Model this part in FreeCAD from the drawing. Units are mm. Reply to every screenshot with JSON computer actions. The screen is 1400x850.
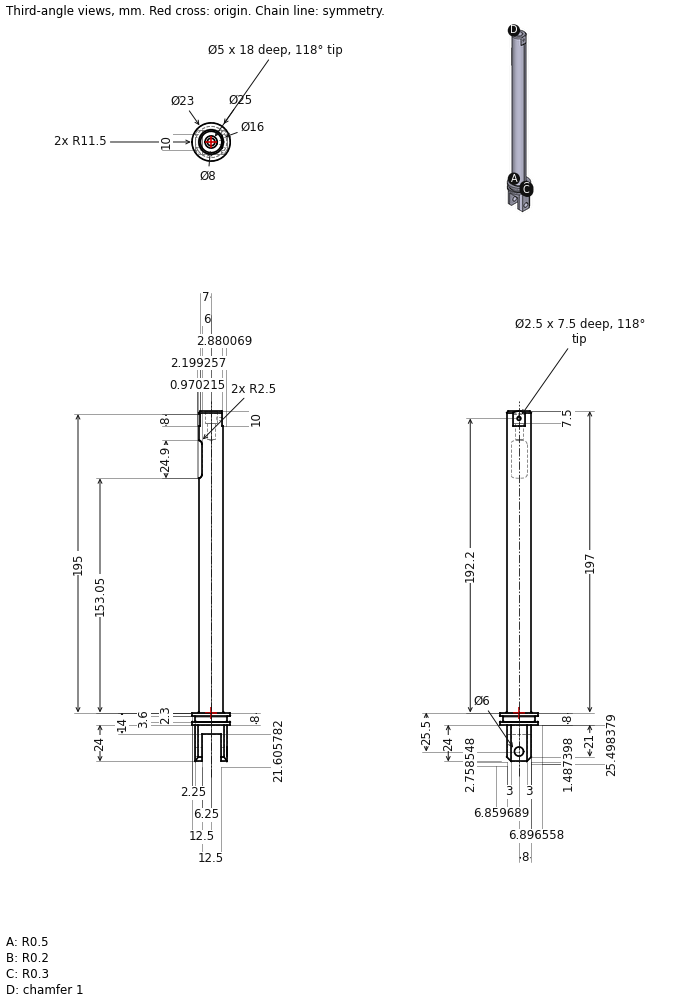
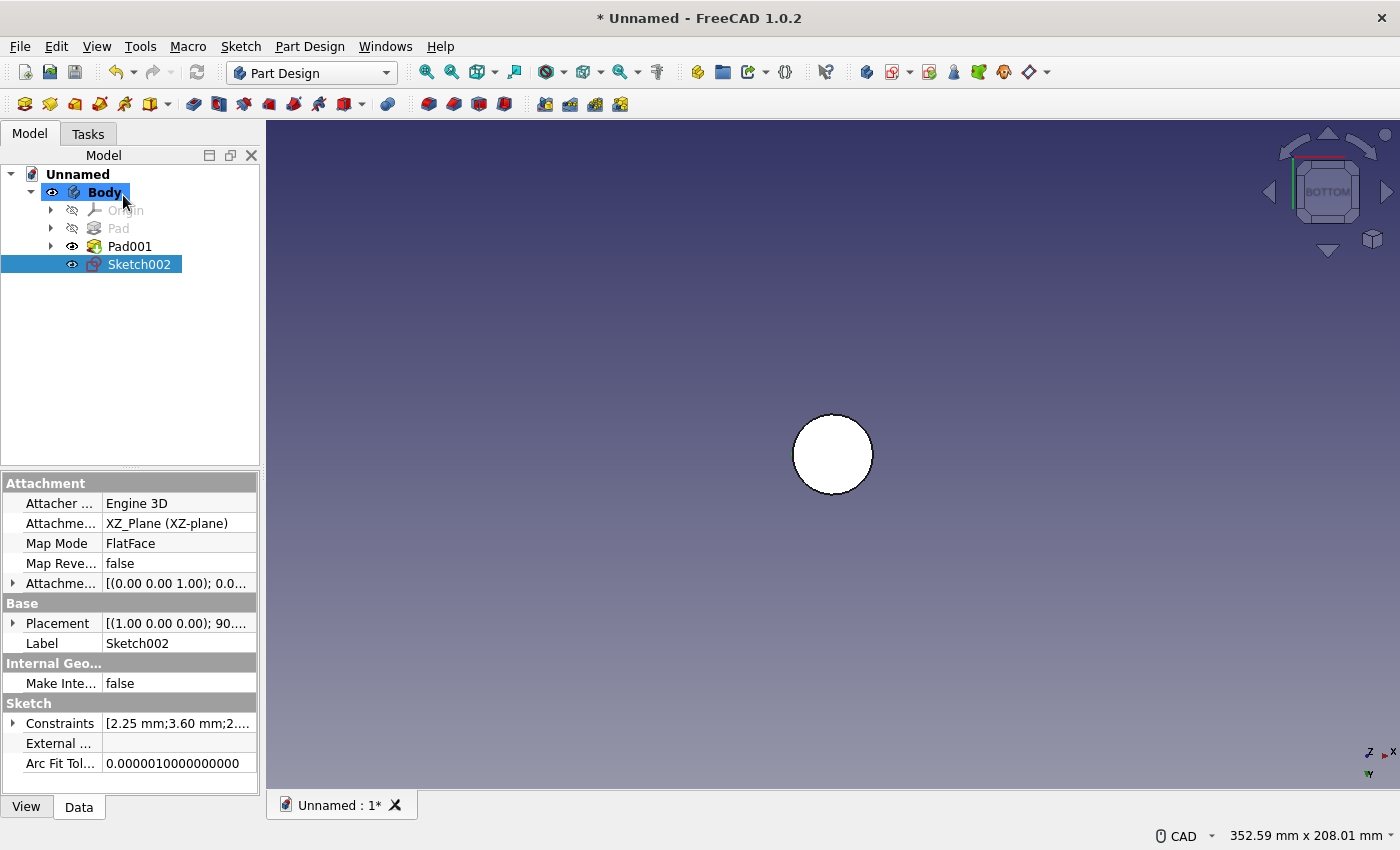
{"action": "left_click", "coordinate": [244, 104]}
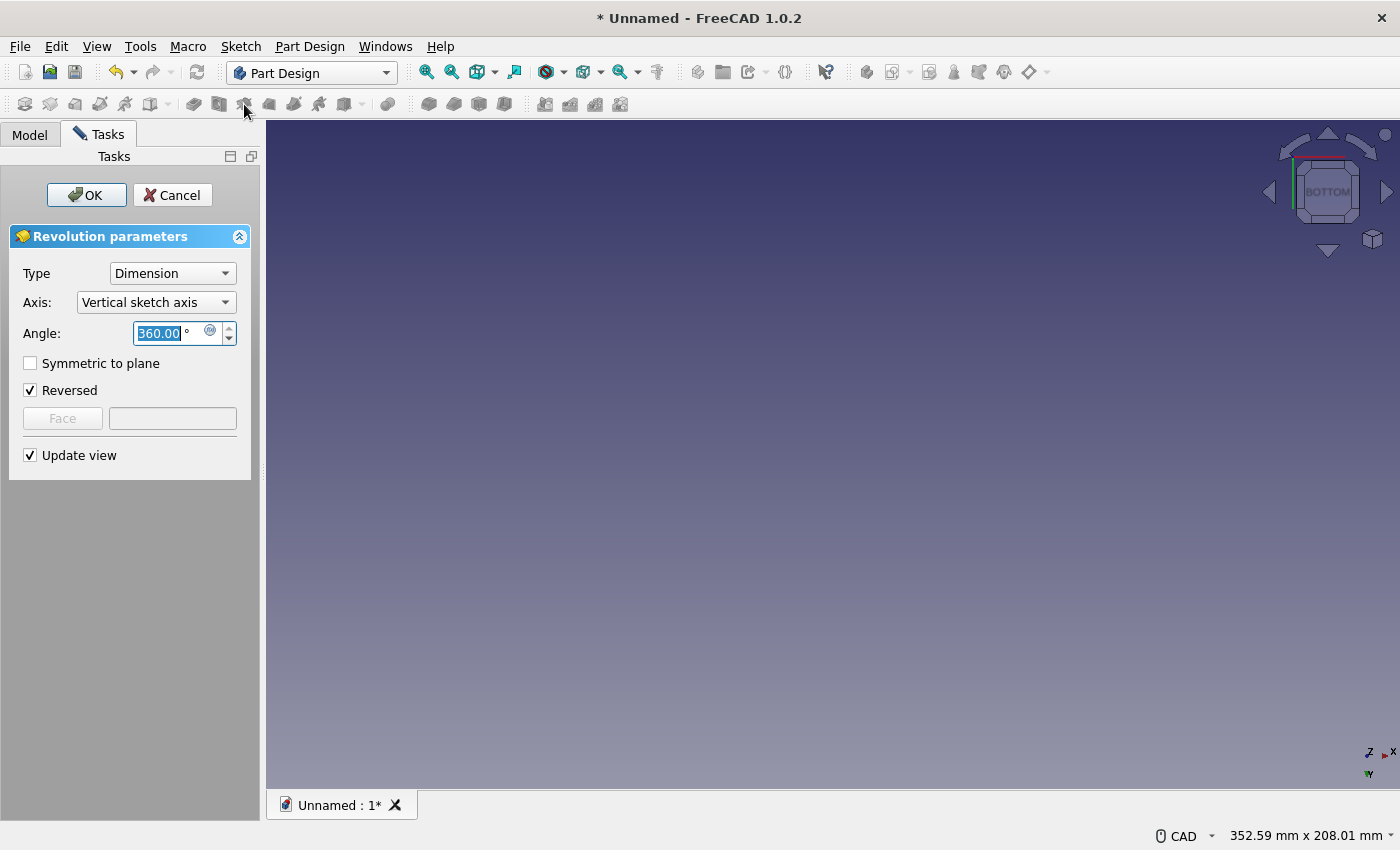
{"action": "left_click", "coordinate": [87, 195]}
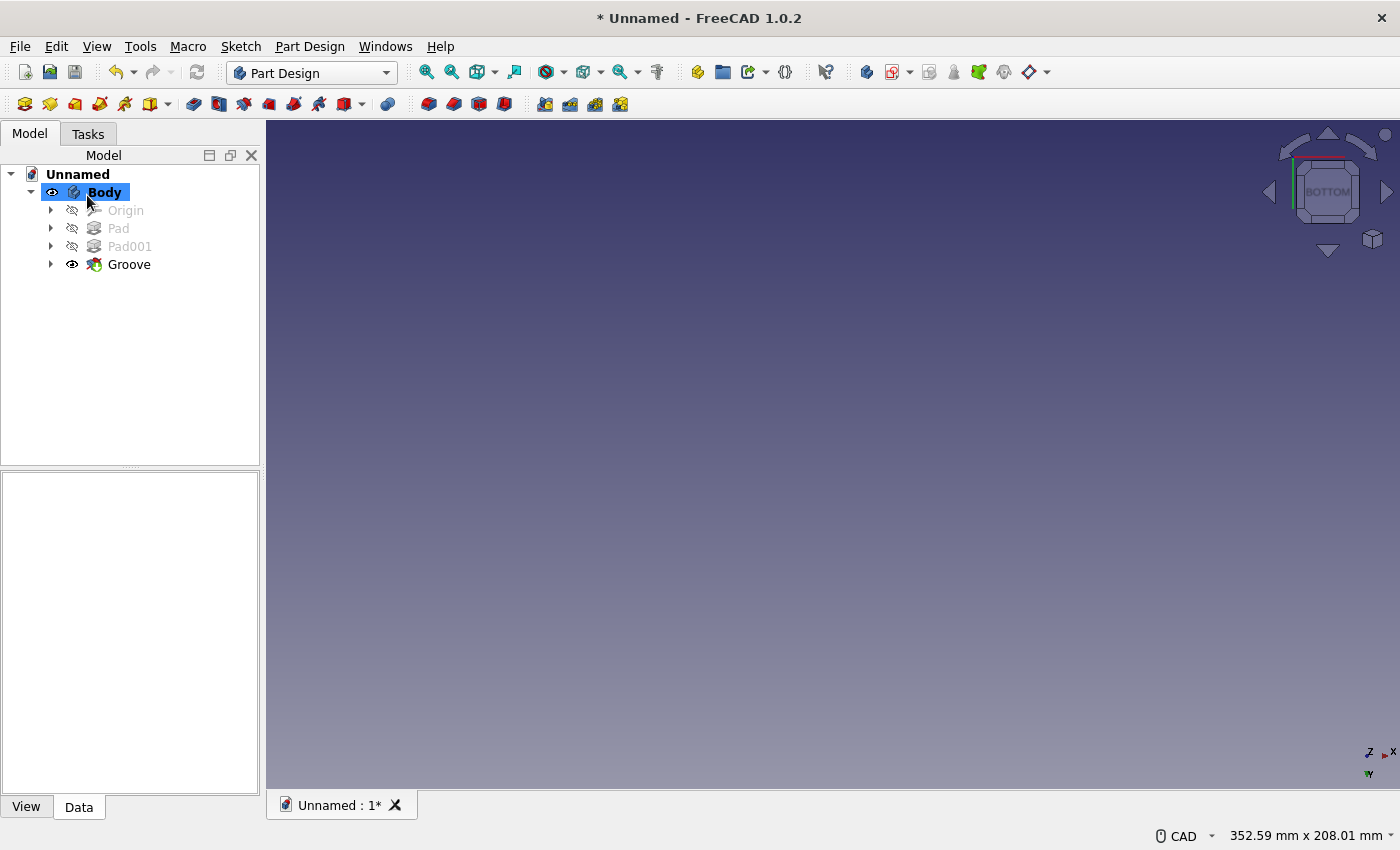
{"action": "left_click", "coordinate": [427, 72]}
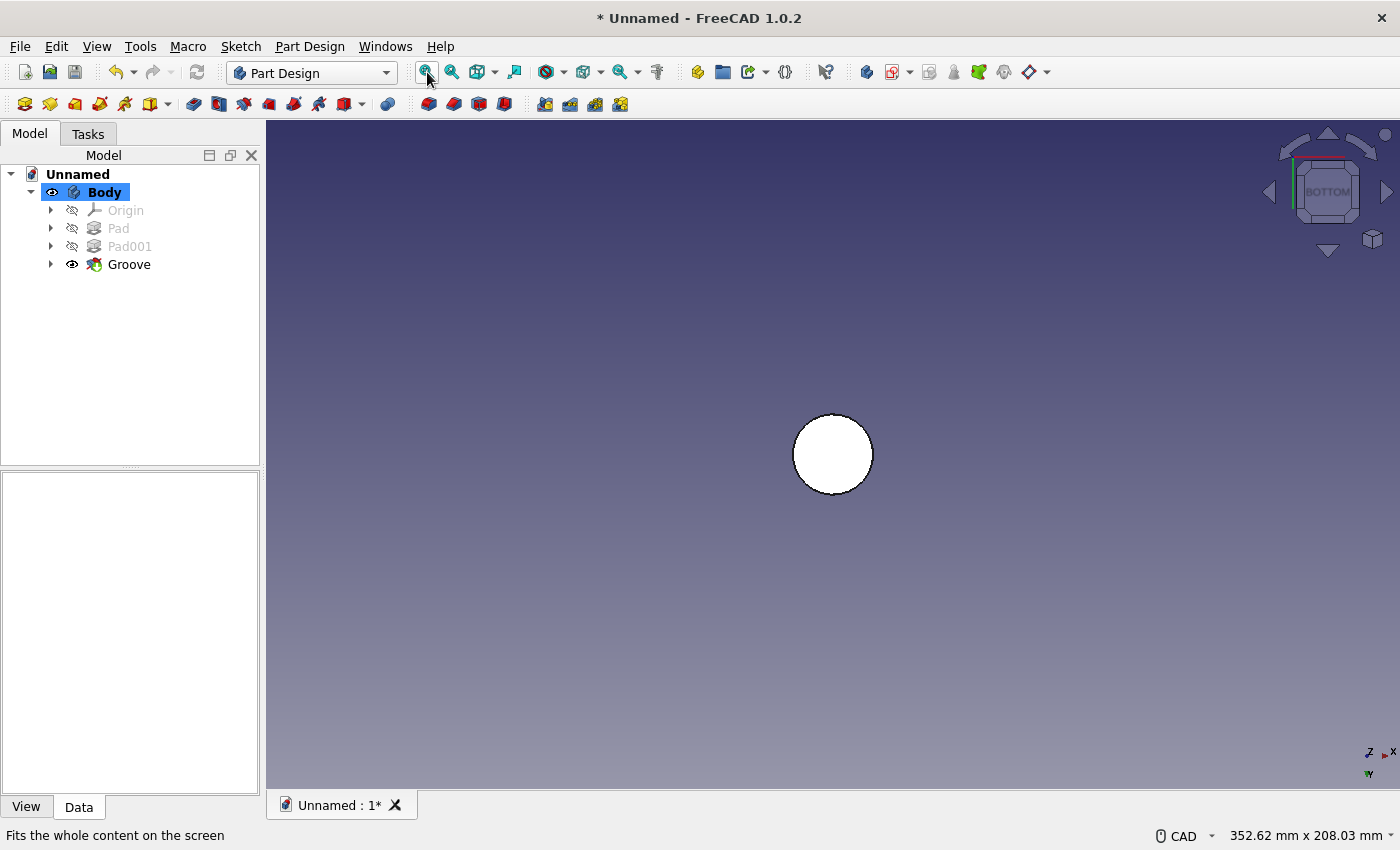
{"action": "left_click", "coordinate": [833, 453]}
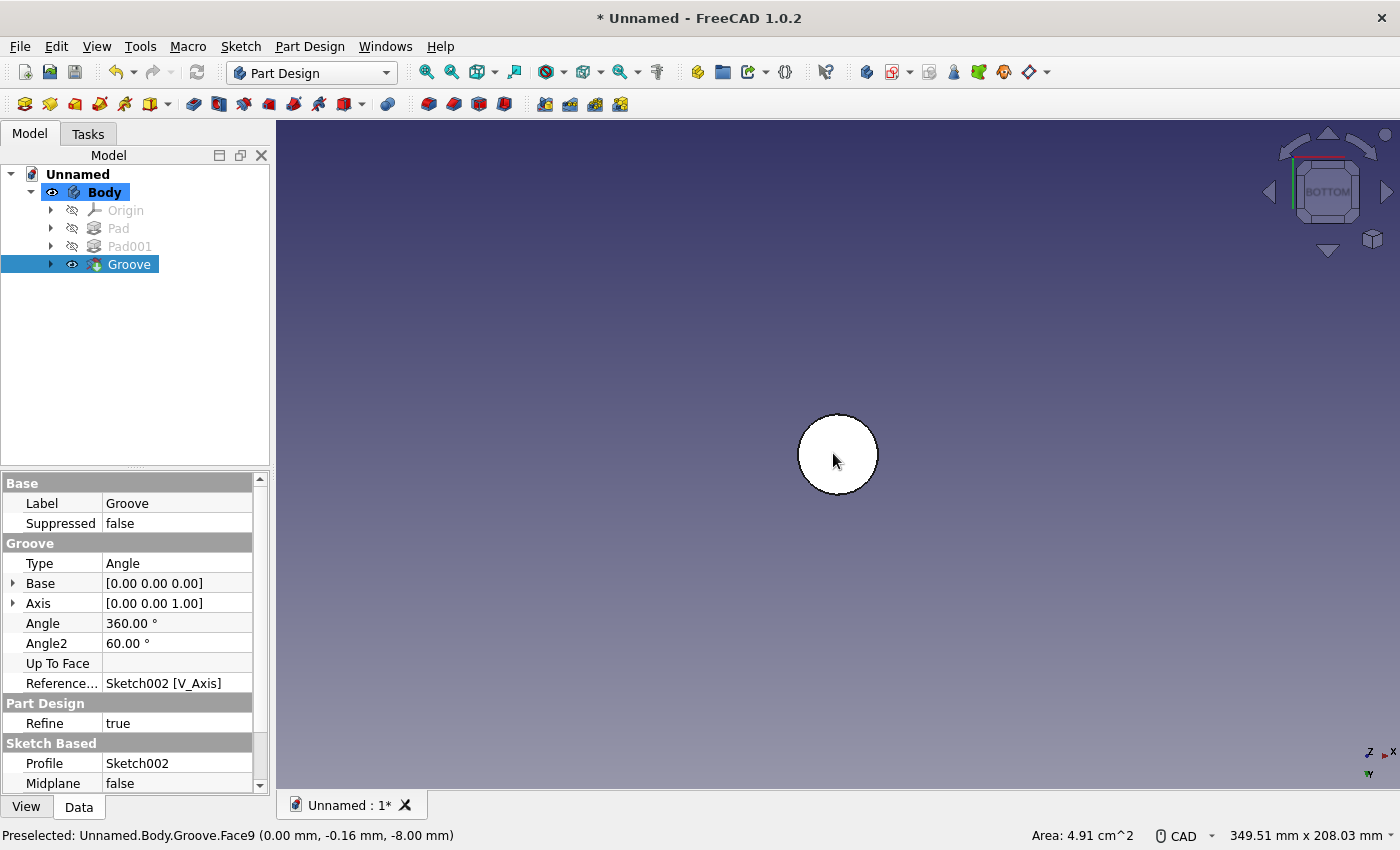
{"action": "left_click", "coordinate": [892, 72]}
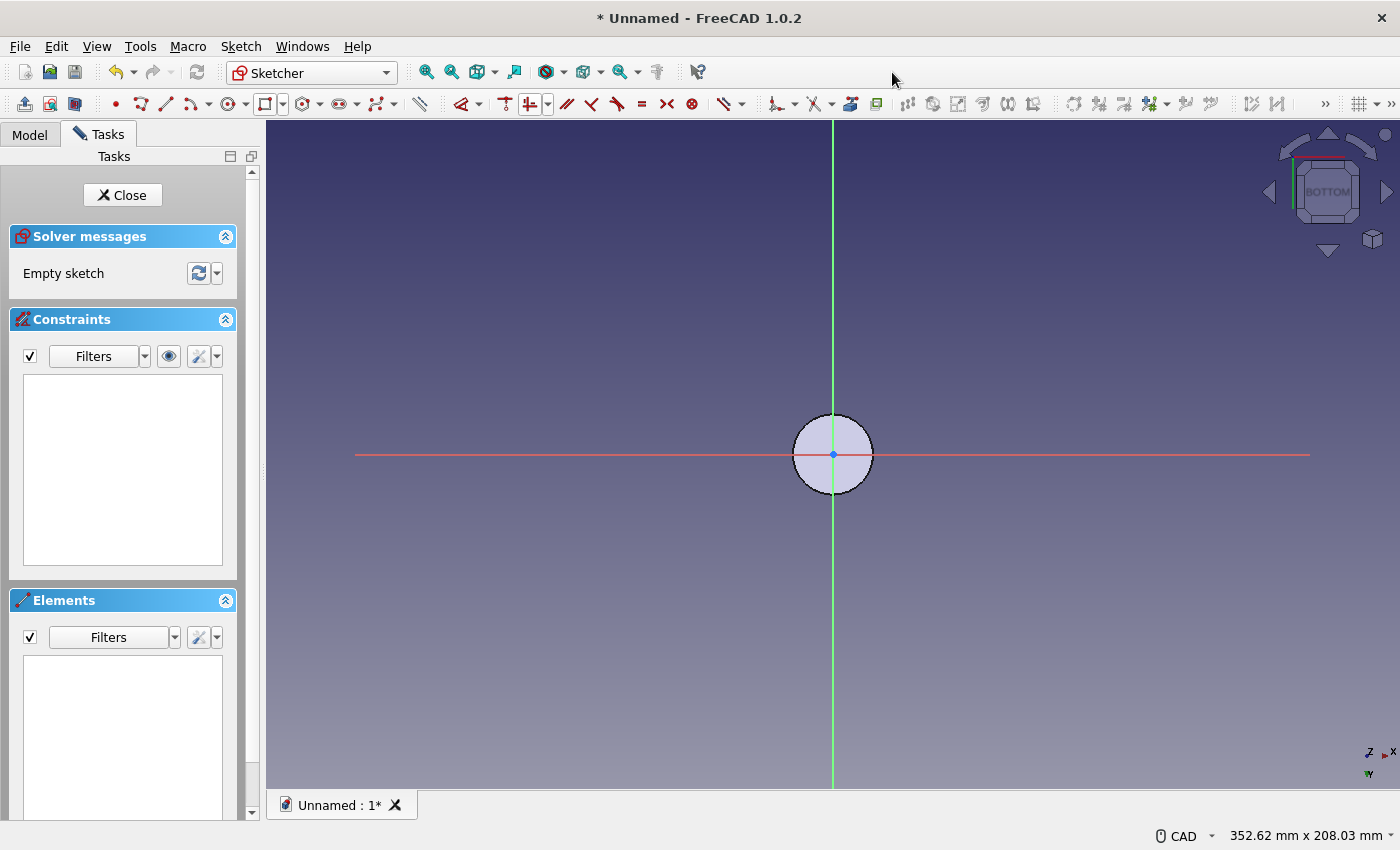
{"action": "scroll", "coordinate": [847, 455], "scroll_direction": "up", "scroll_amount": 9}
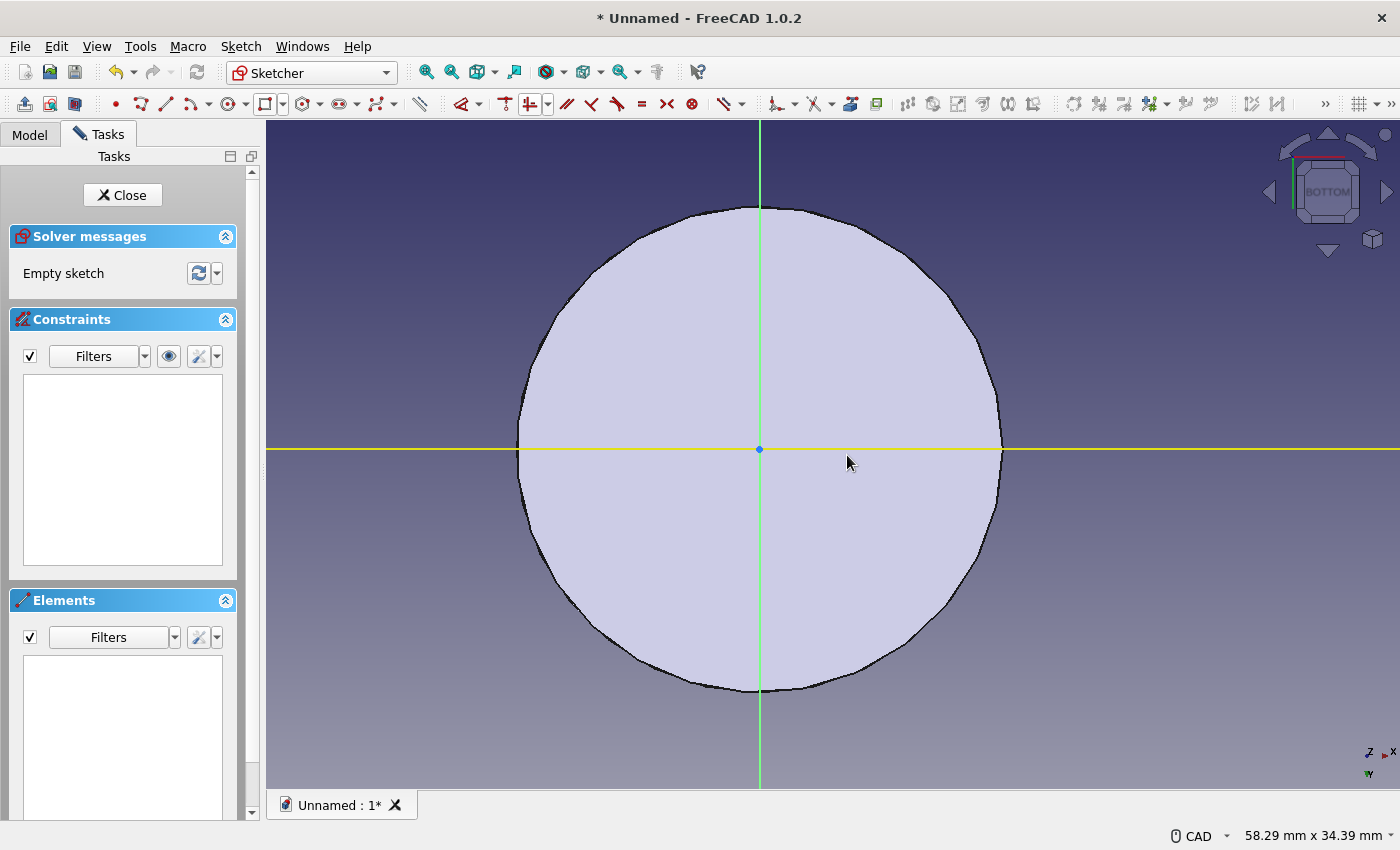
{"action": "left_click", "coordinate": [228, 104]}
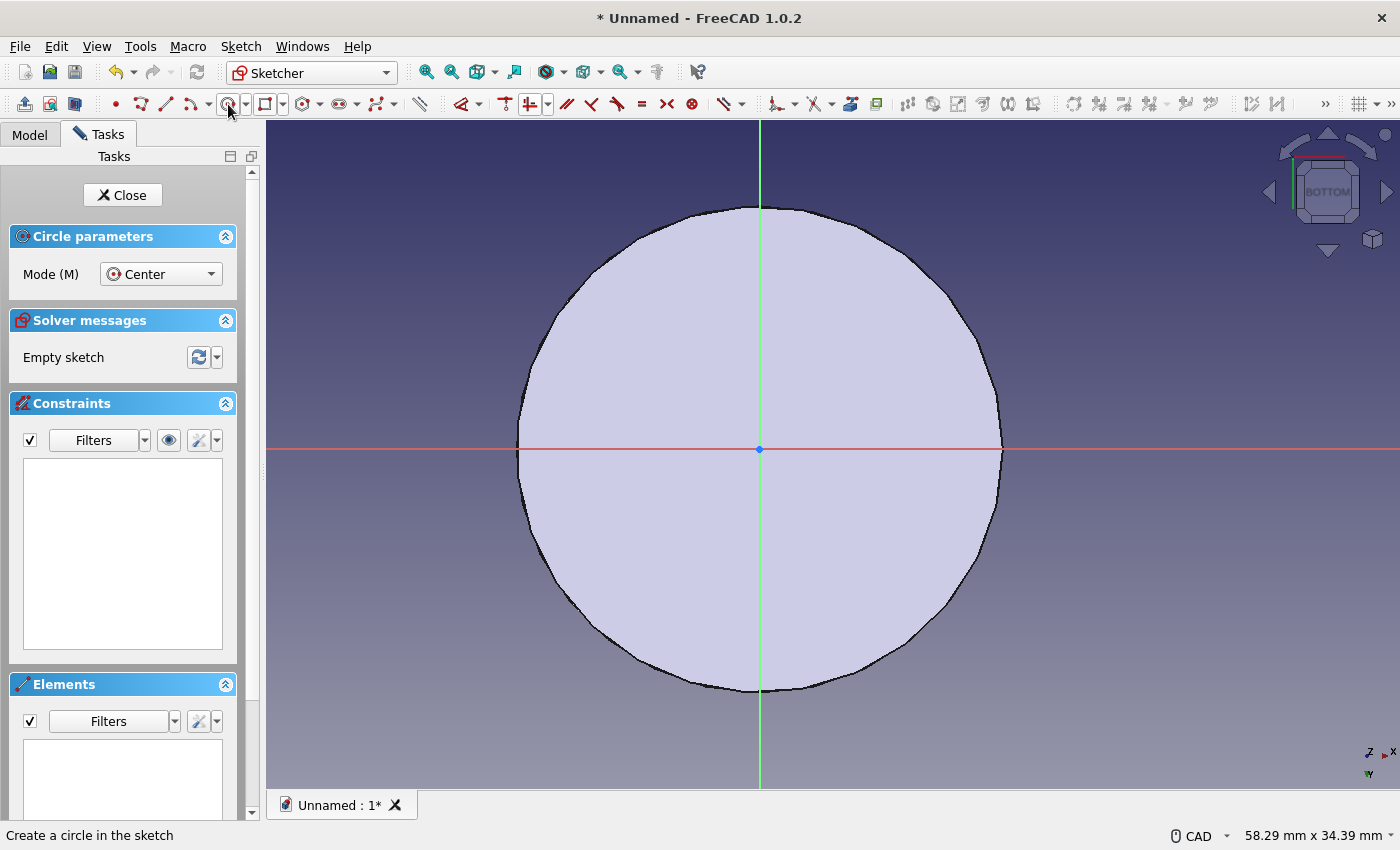
{"action": "left_click", "coordinate": [760, 449]}
{"action": "mouse_move", "coordinate": [918, 291]}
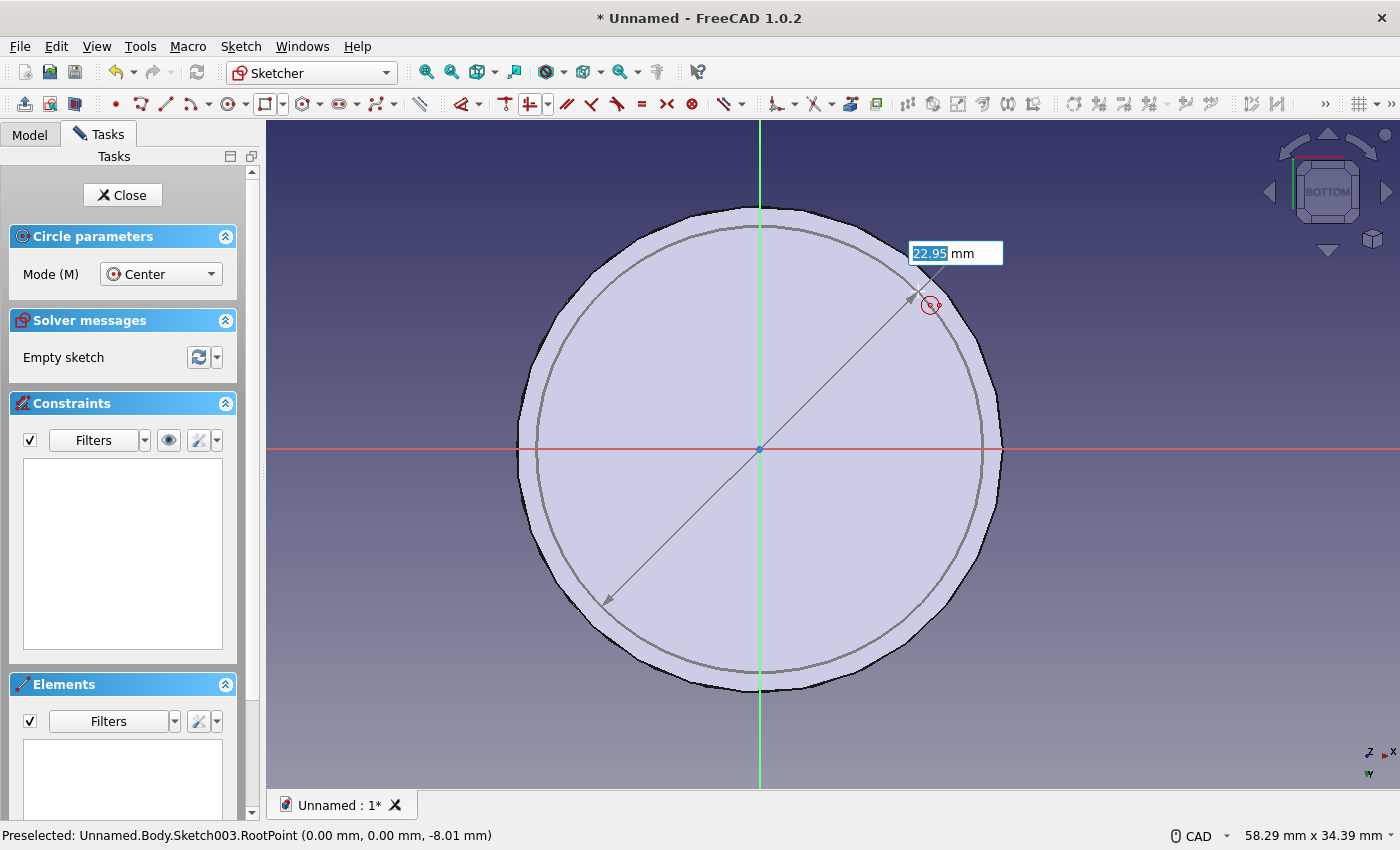
{"action": "type", "text": "23"}
{"action": "key", "text": "Return"}
{"action": "key", "text": "Escape"}